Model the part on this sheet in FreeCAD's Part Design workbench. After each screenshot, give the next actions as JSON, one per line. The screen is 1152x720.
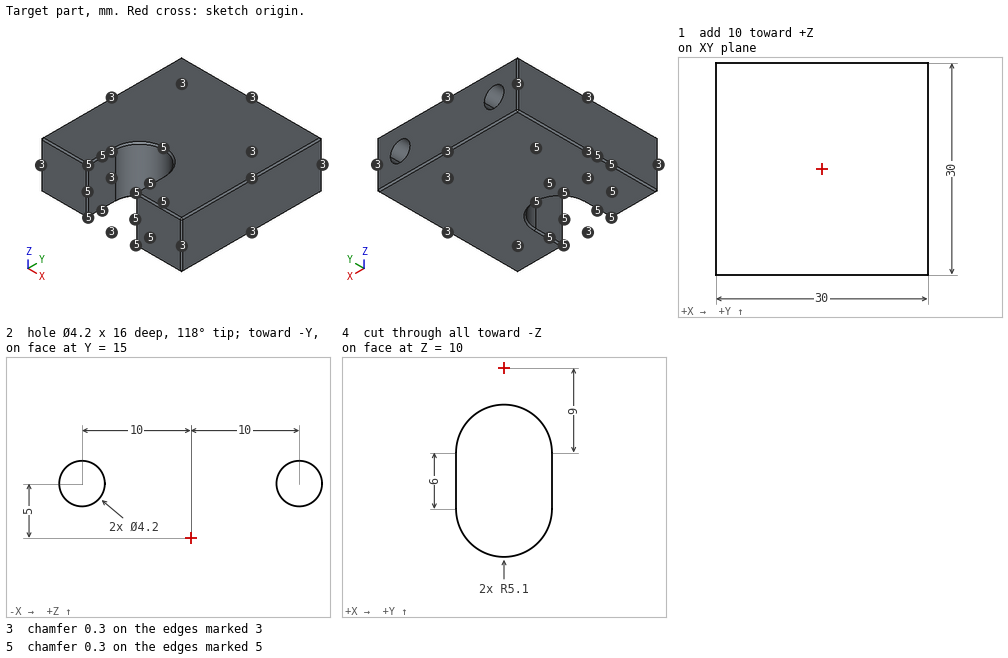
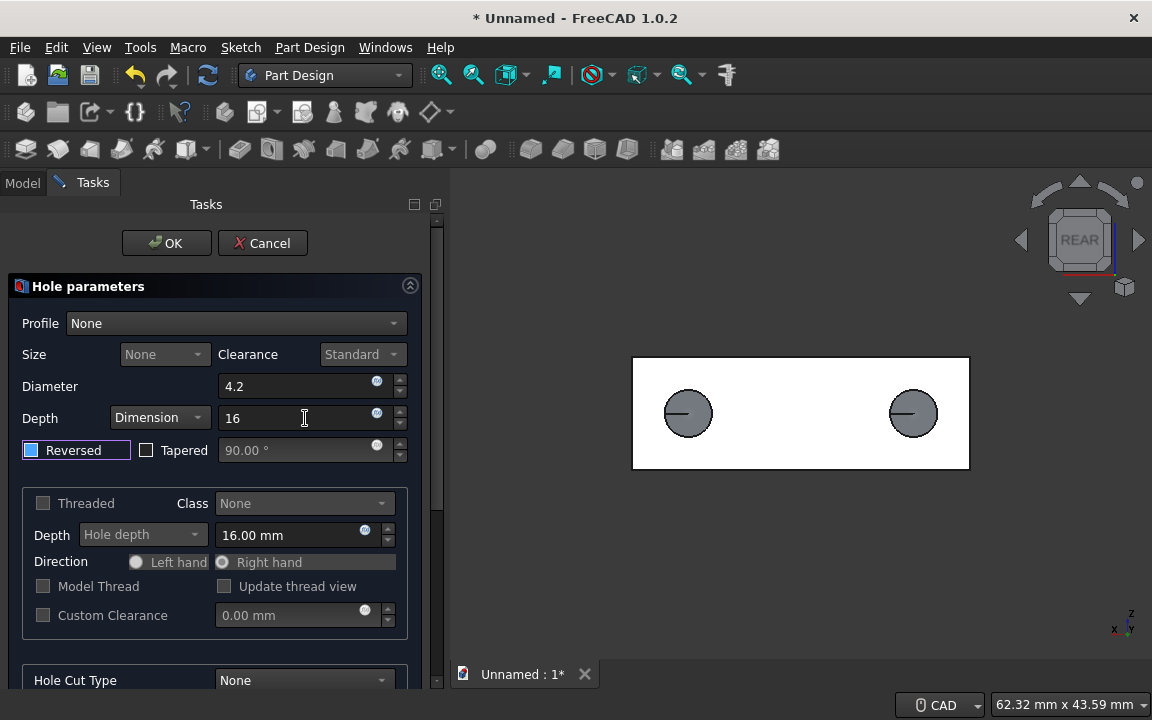
{"action": "left_click", "coordinate": [167, 243]}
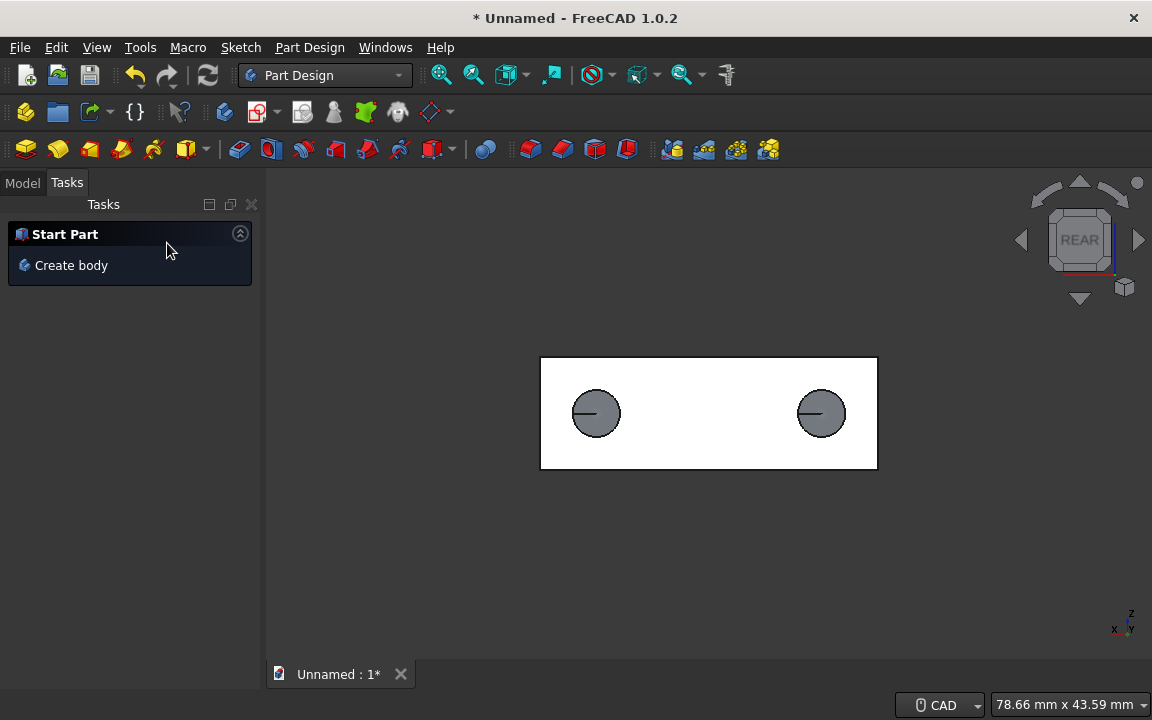
{"action": "left_click", "coordinate": [442, 76]}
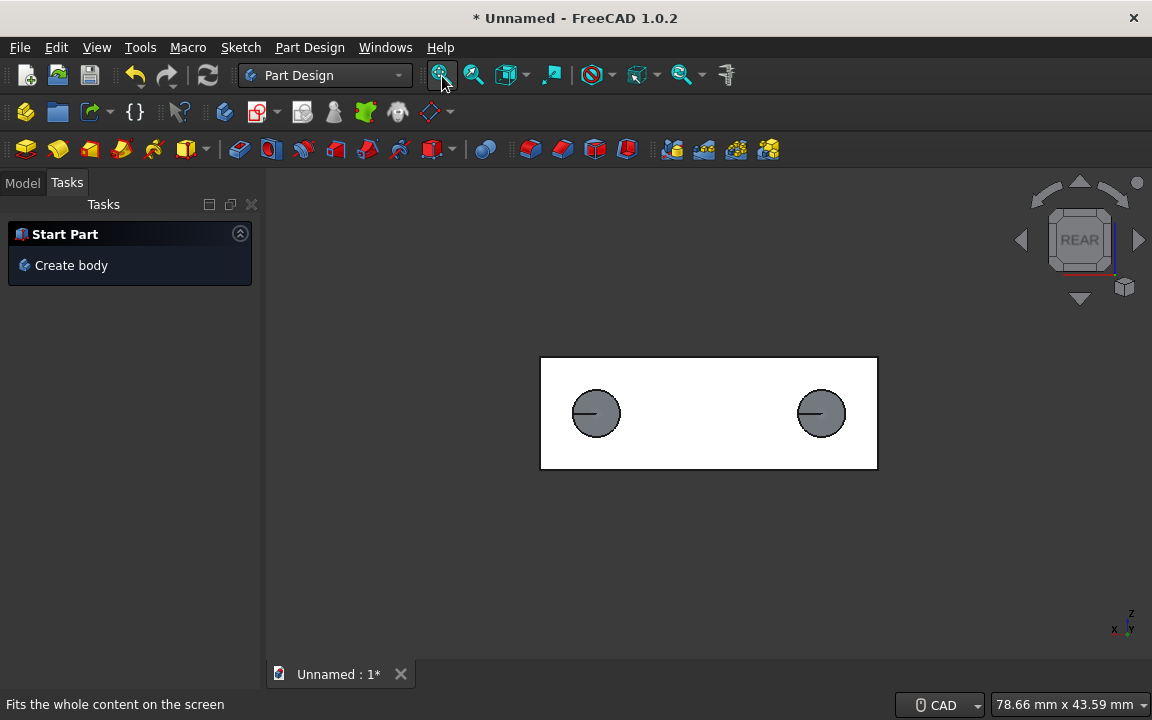
{"action": "left_click", "coordinate": [878, 412]}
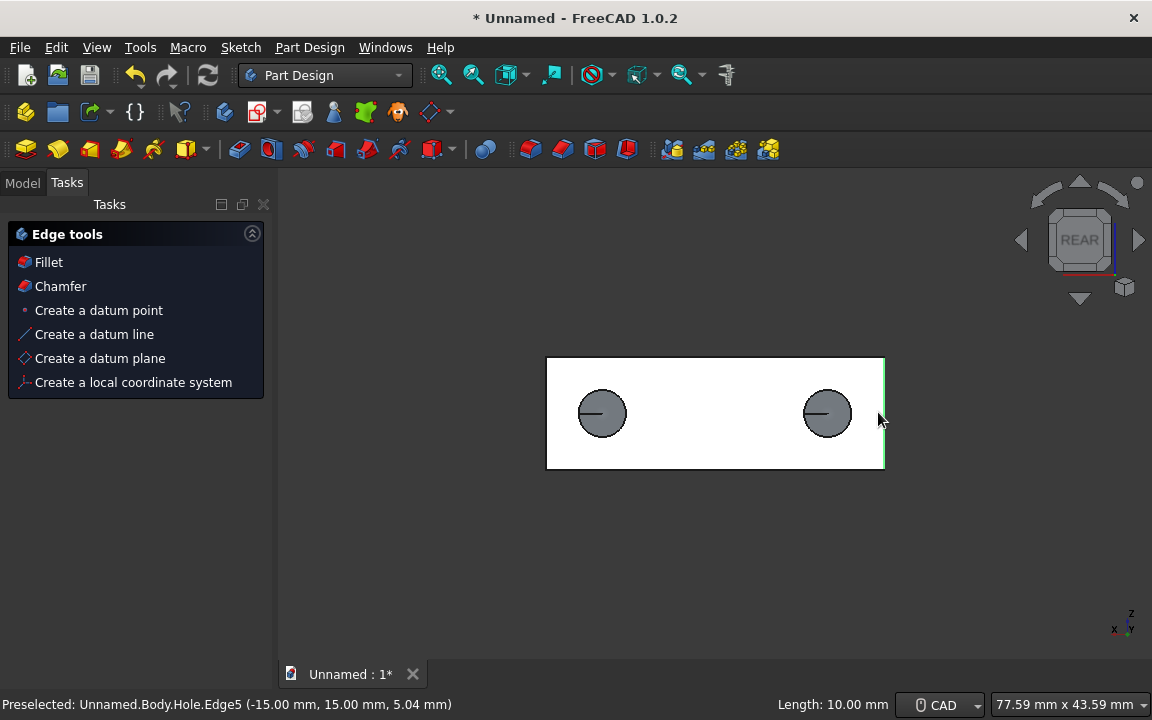
{"action": "key", "text": "0"}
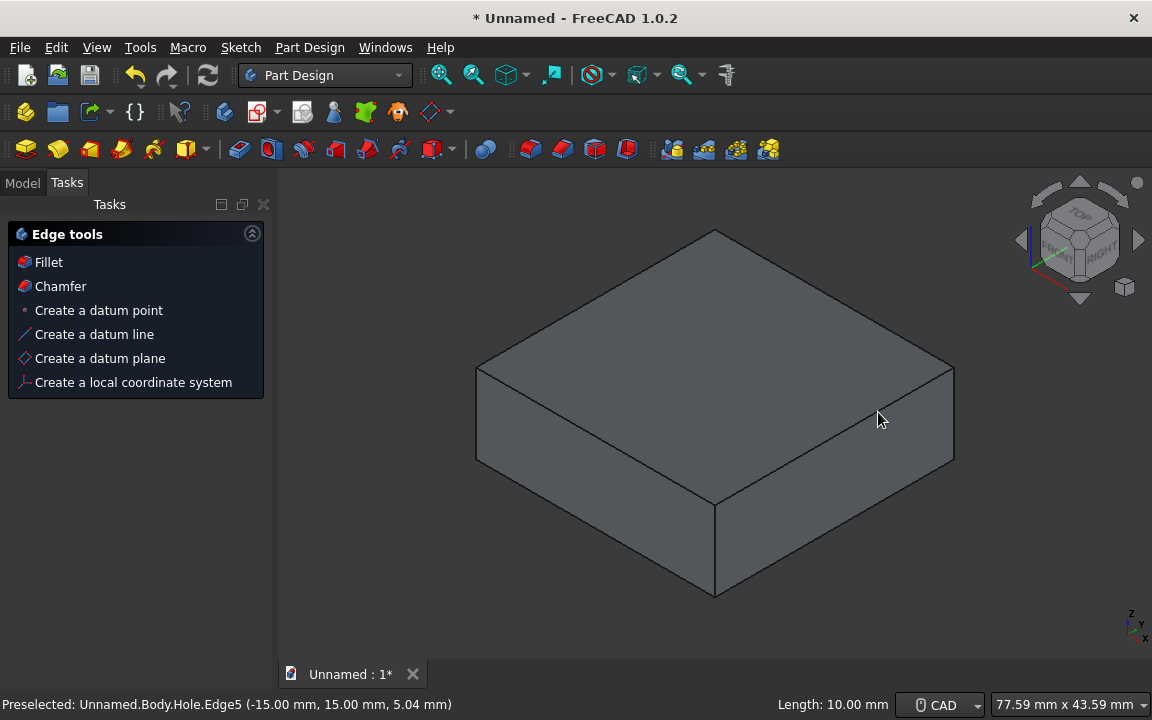
{"action": "left_click", "coordinate": [715, 367], "text": "ctrl"}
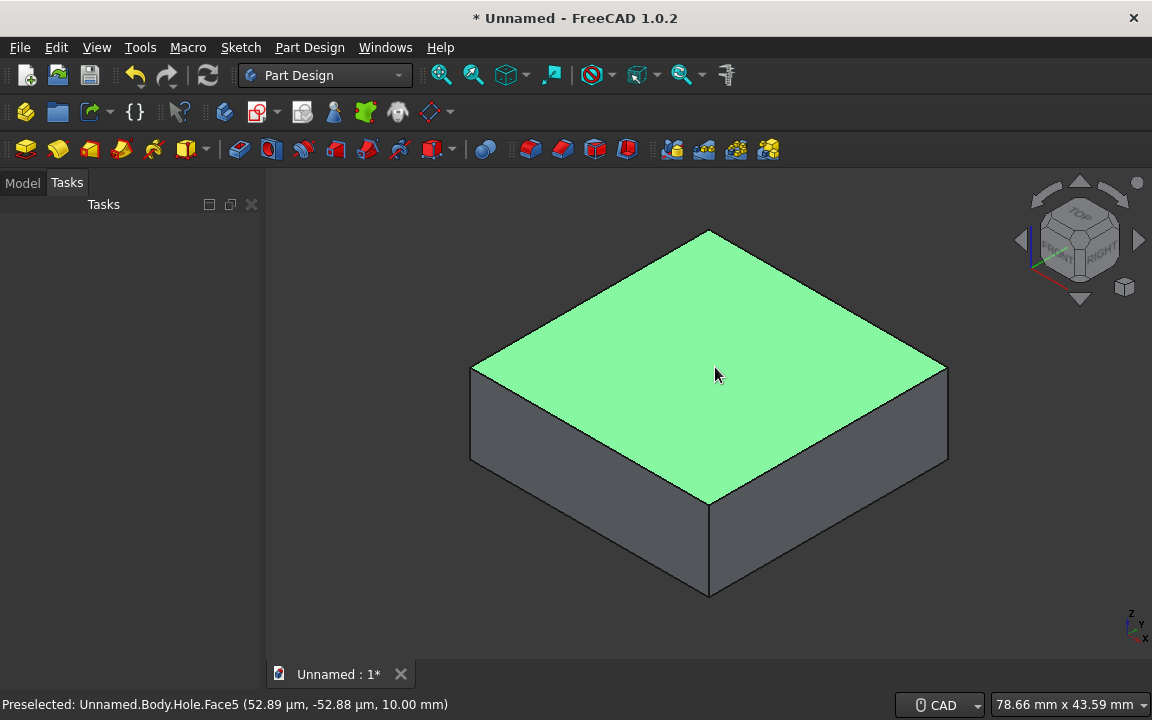
{"action": "left_click", "coordinate": [709, 550], "text": "ctrl"}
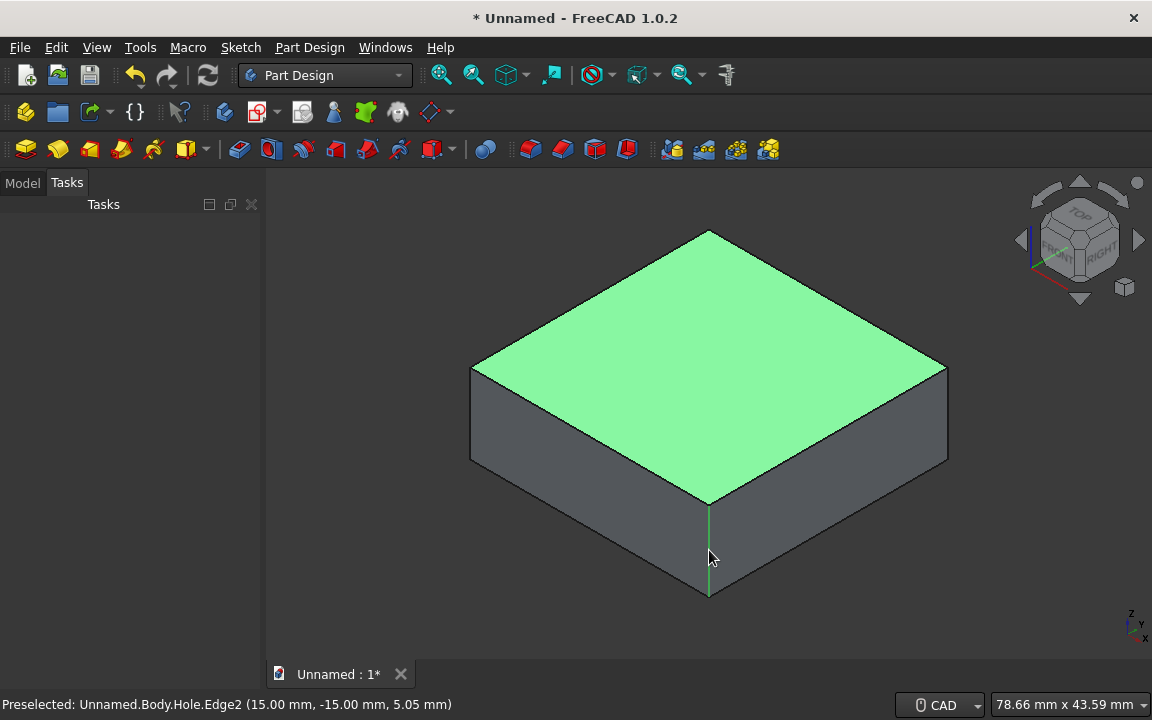
{"action": "key", "text": "2"}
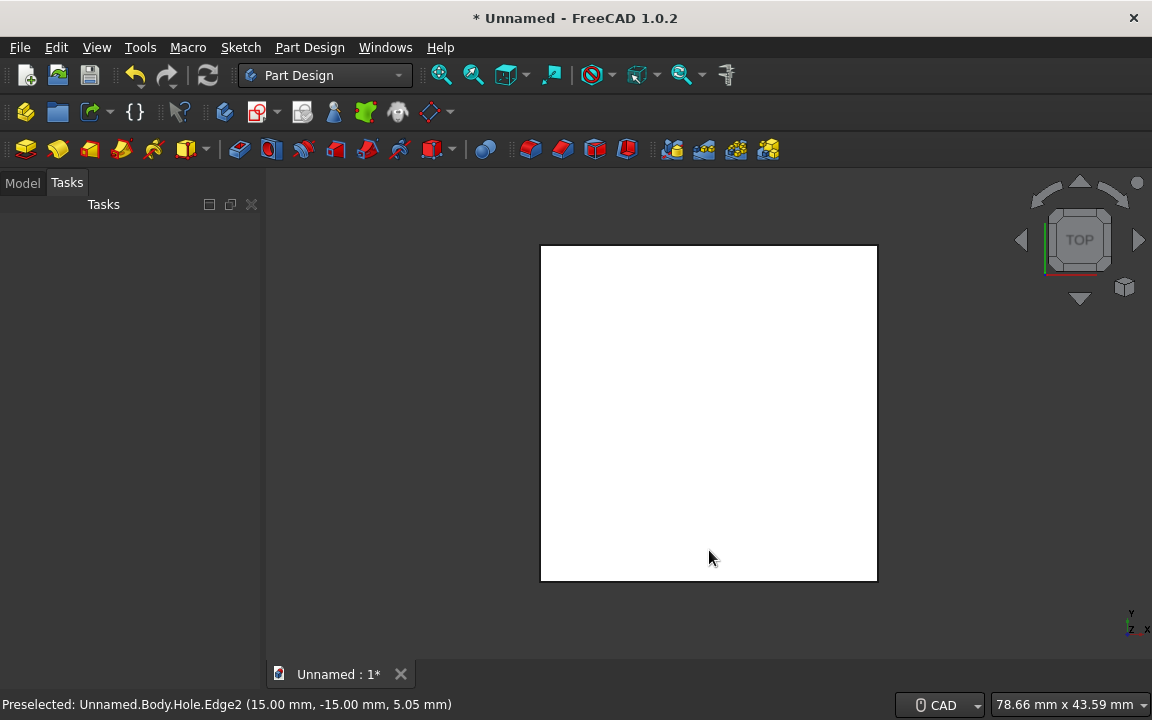
{"action": "key", "text": "1"}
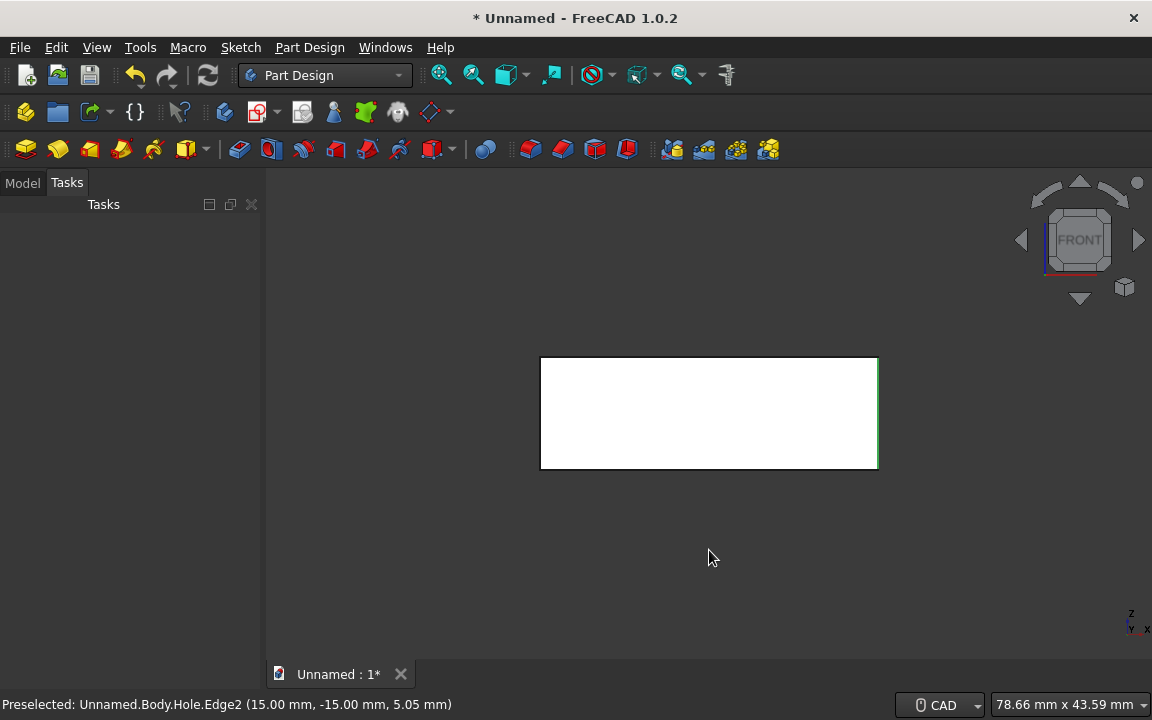
{"action": "left_click", "coordinate": [442, 76]}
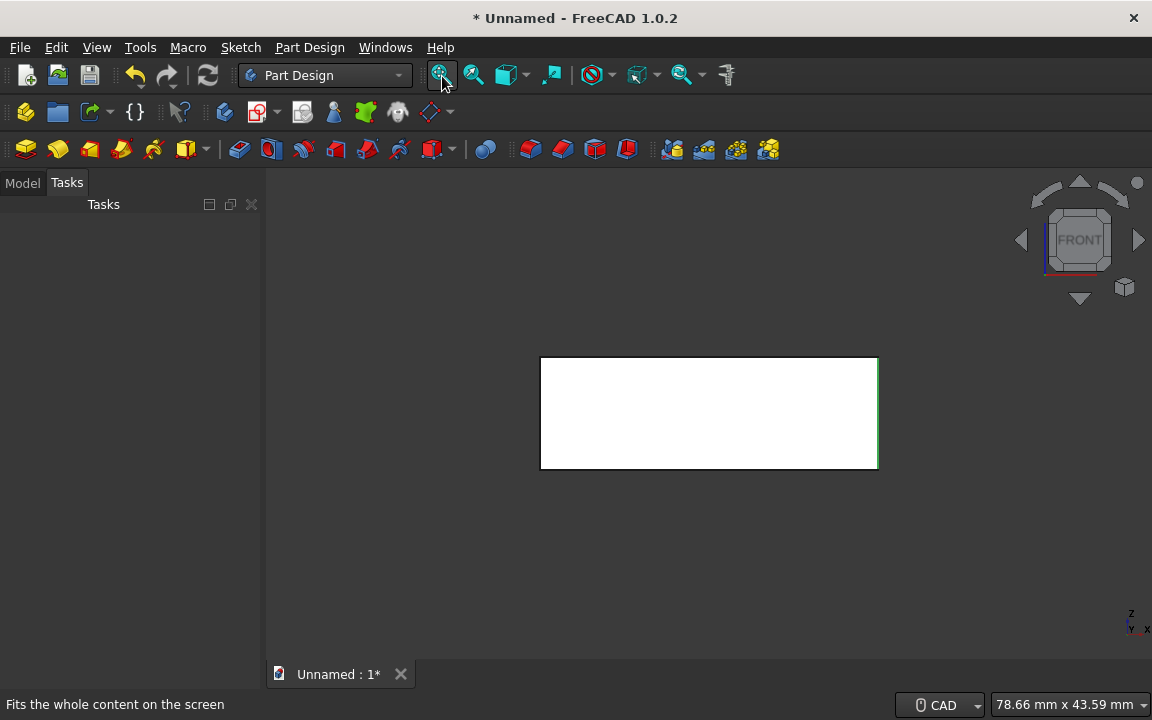
{"action": "left_click", "coordinate": [540, 413], "text": "ctrl"}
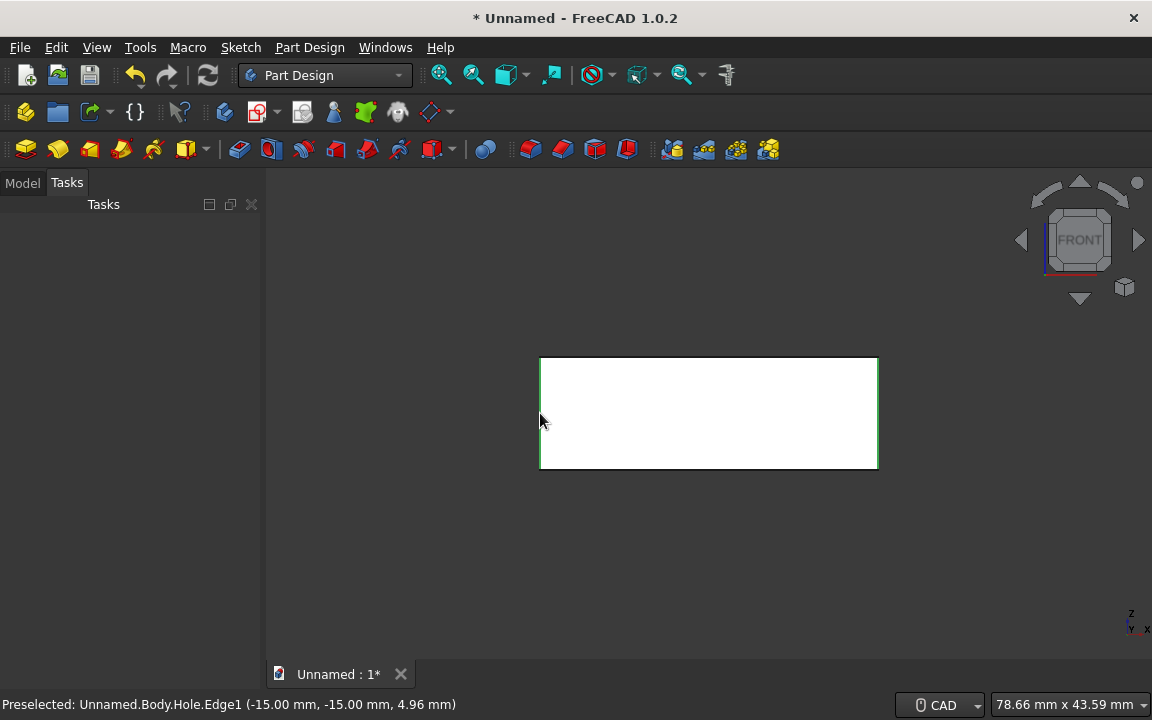
{"action": "key", "text": "3"}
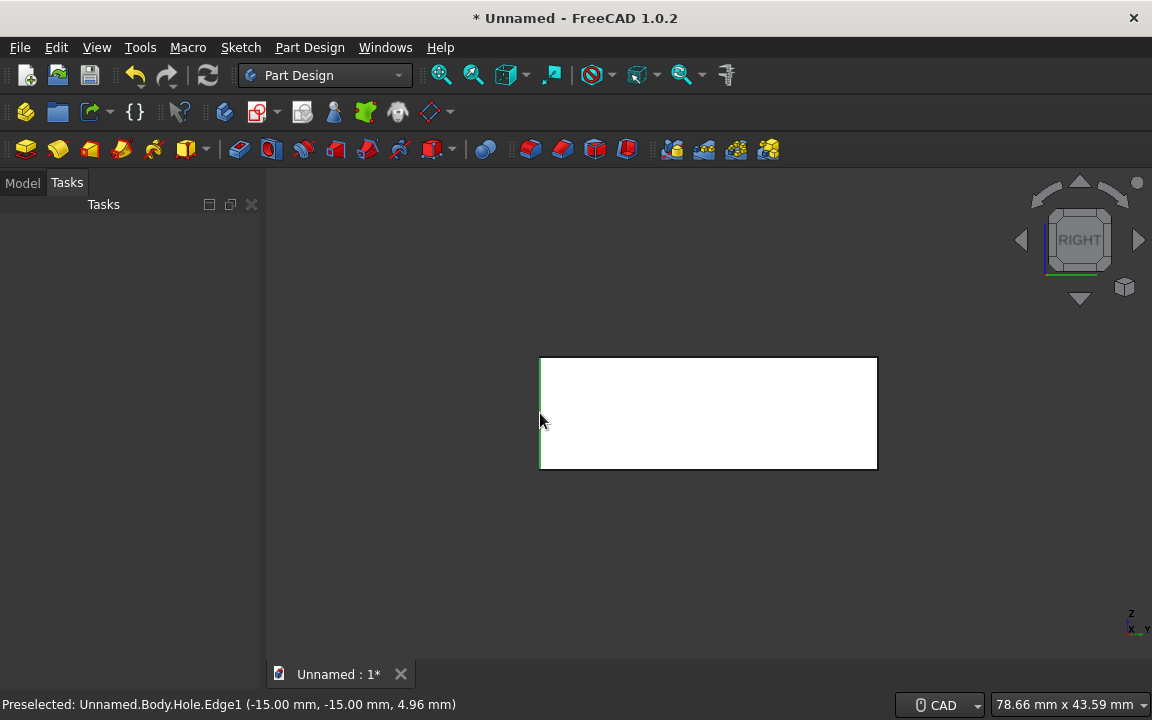
{"action": "left_click", "coordinate": [442, 76]}